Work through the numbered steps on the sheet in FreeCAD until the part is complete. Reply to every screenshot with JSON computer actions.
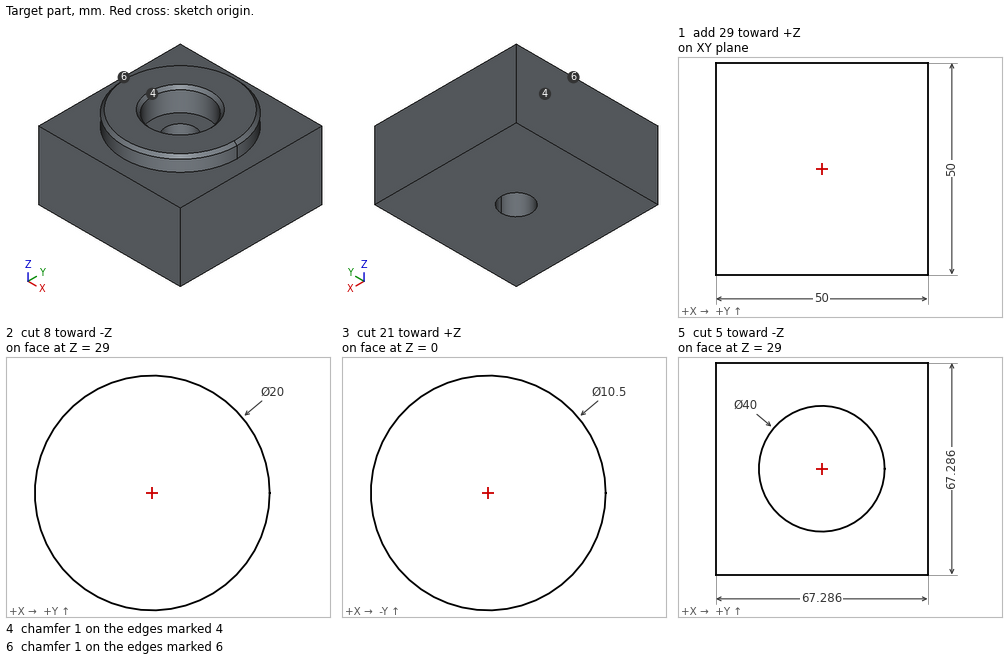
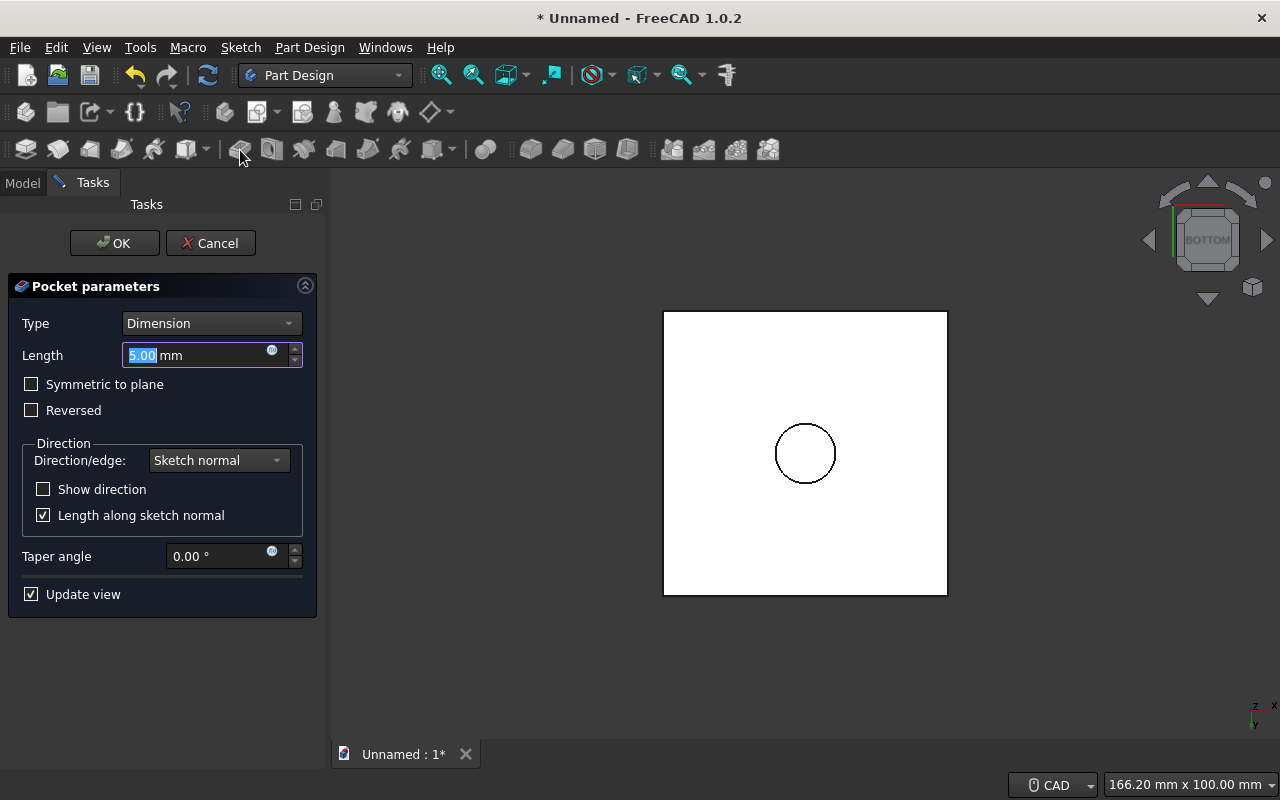
{"action": "type", "text": "21"}
{"action": "key", "text": "Tab"}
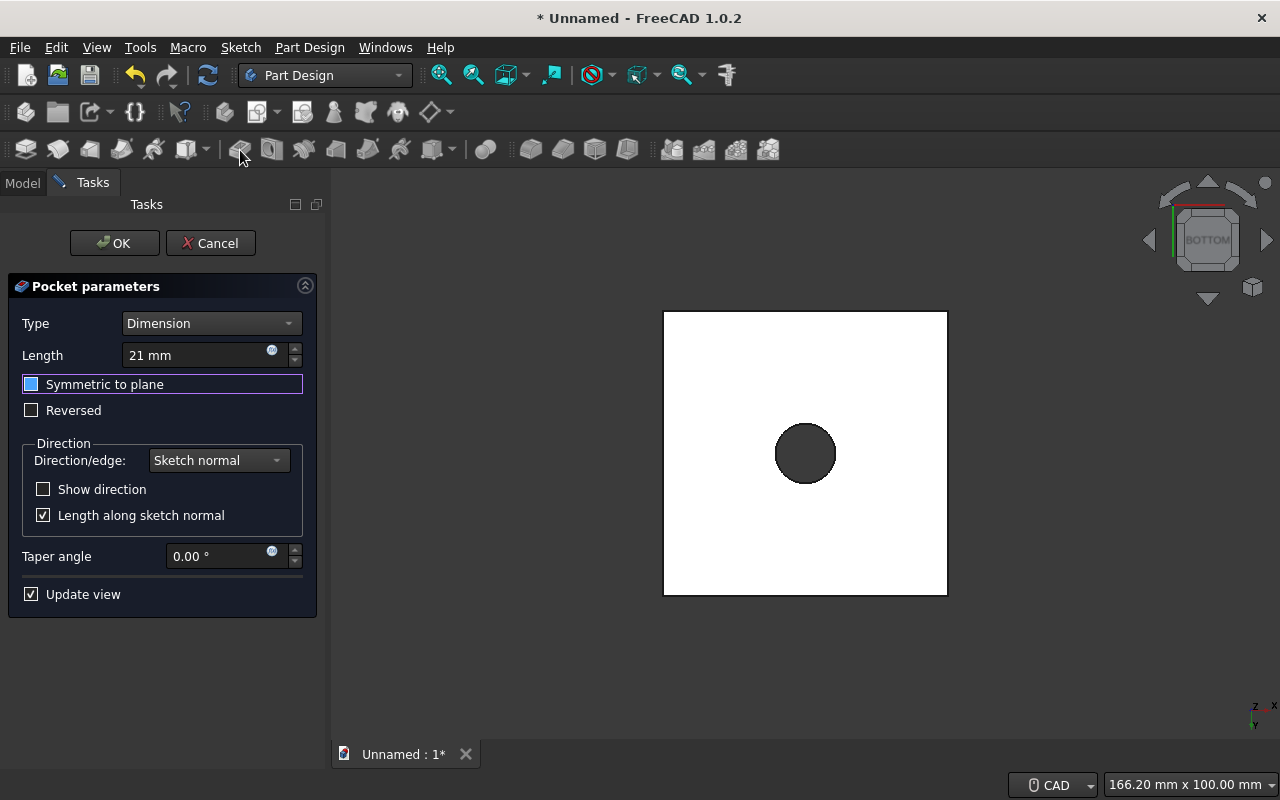
{"action": "left_click", "coordinate": [115, 243]}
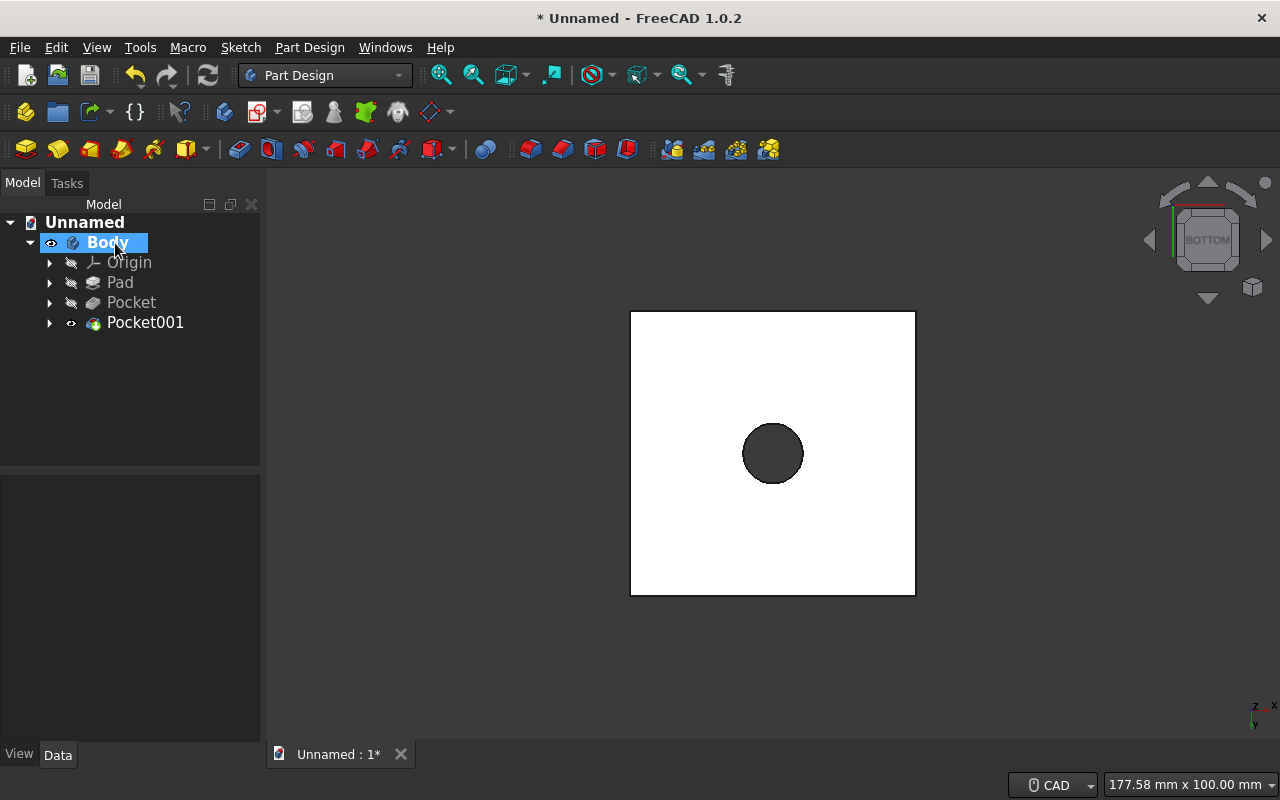
{"action": "key", "text": "0"}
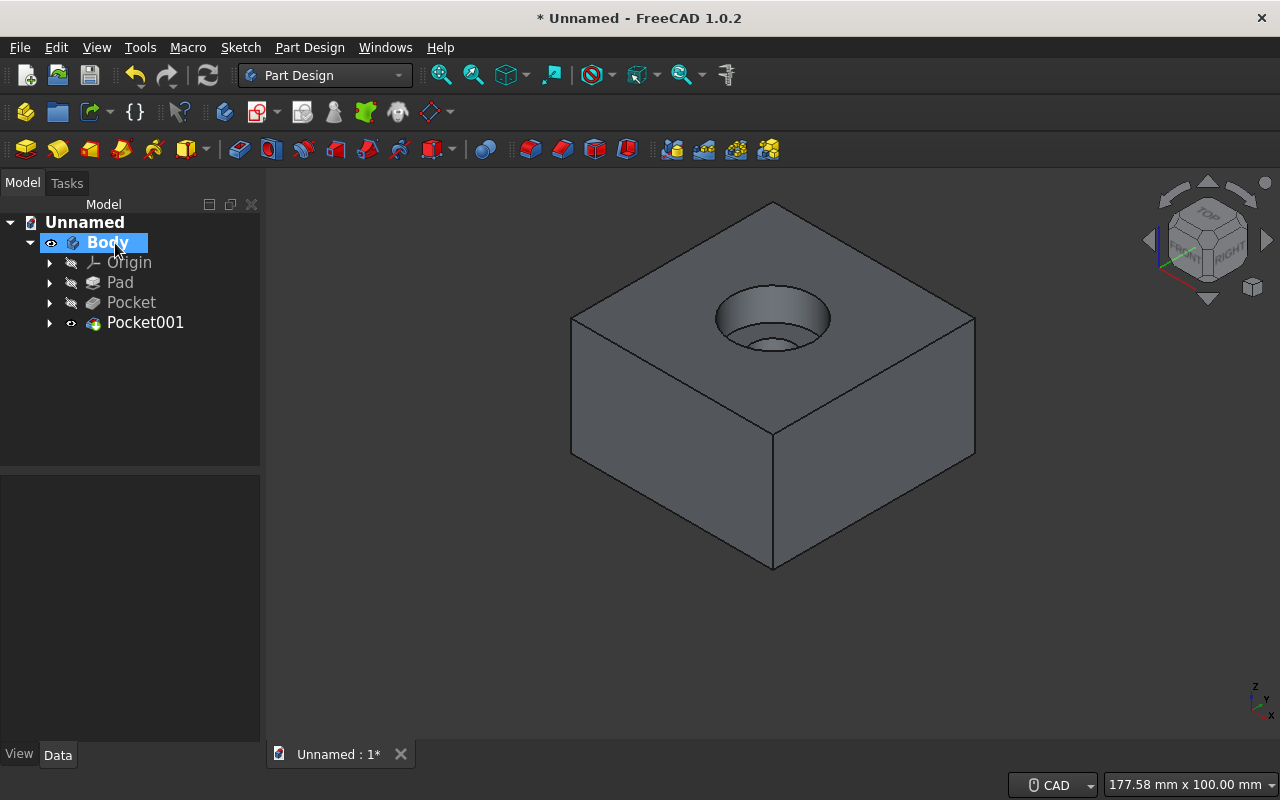
{"action": "left_click", "coordinate": [733, 294]}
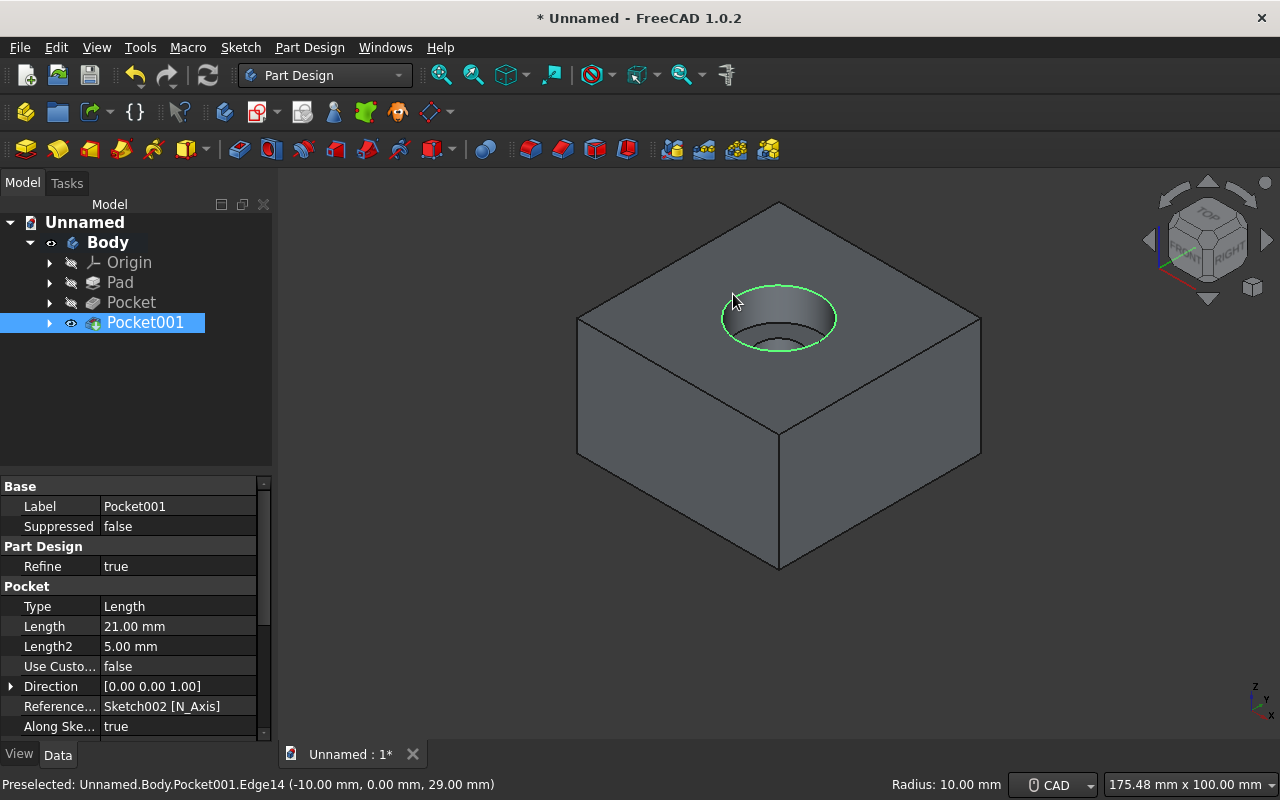
{"action": "left_click", "coordinate": [564, 150]}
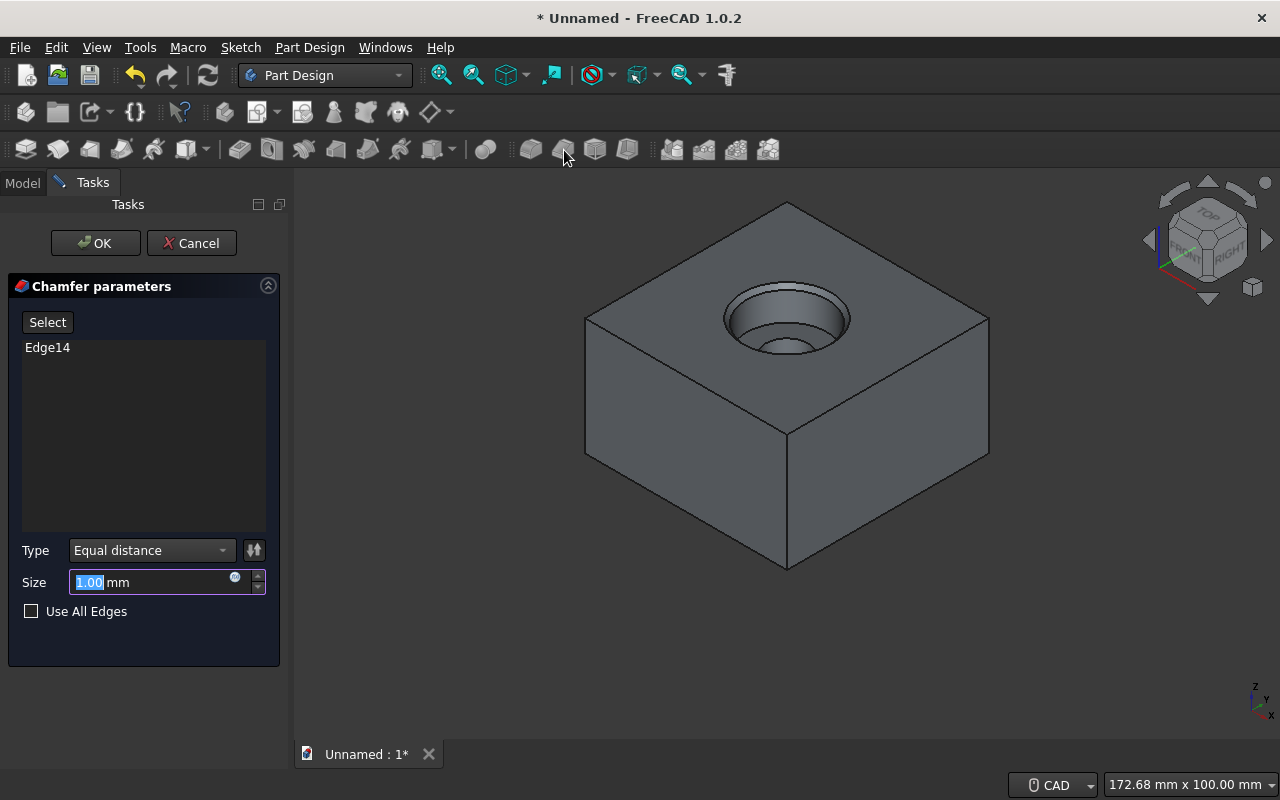
{"action": "type", "text": "1"}
{"action": "key", "text": "Tab"}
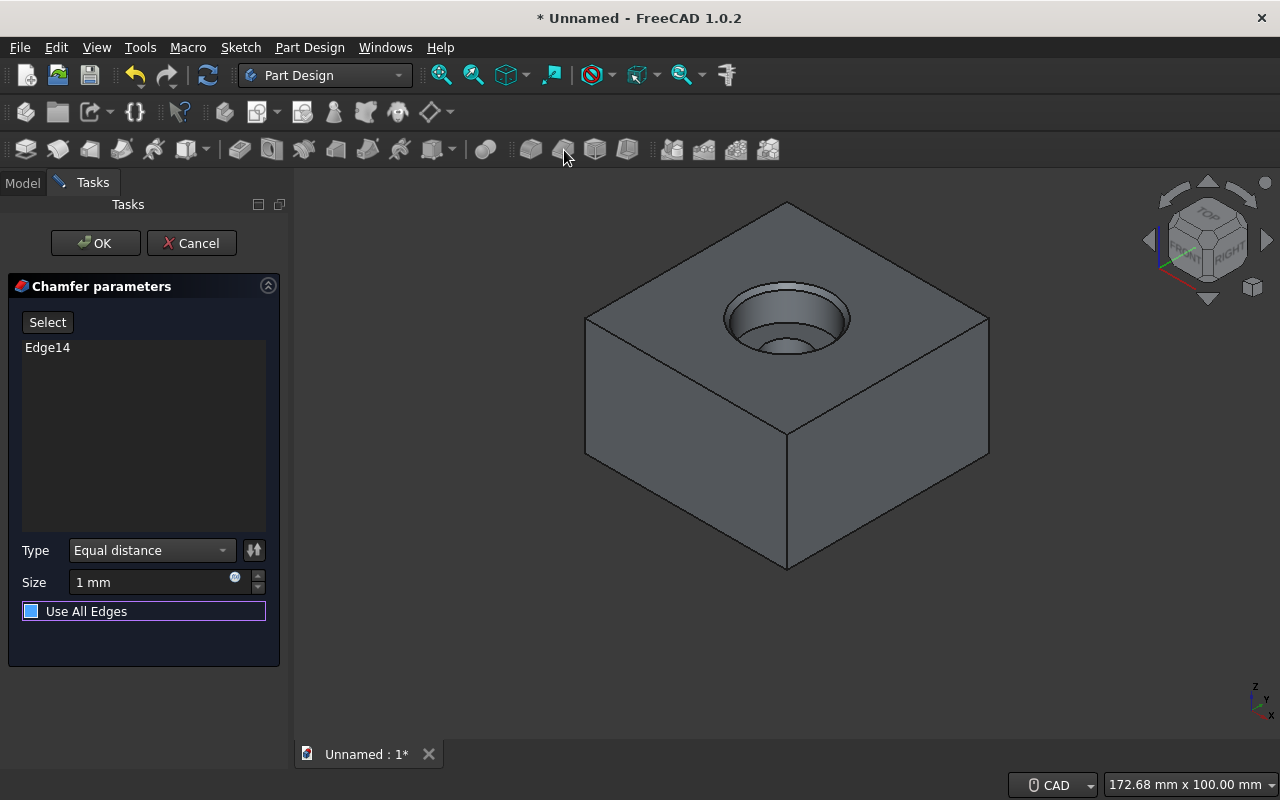
{"action": "left_click", "coordinate": [96, 243]}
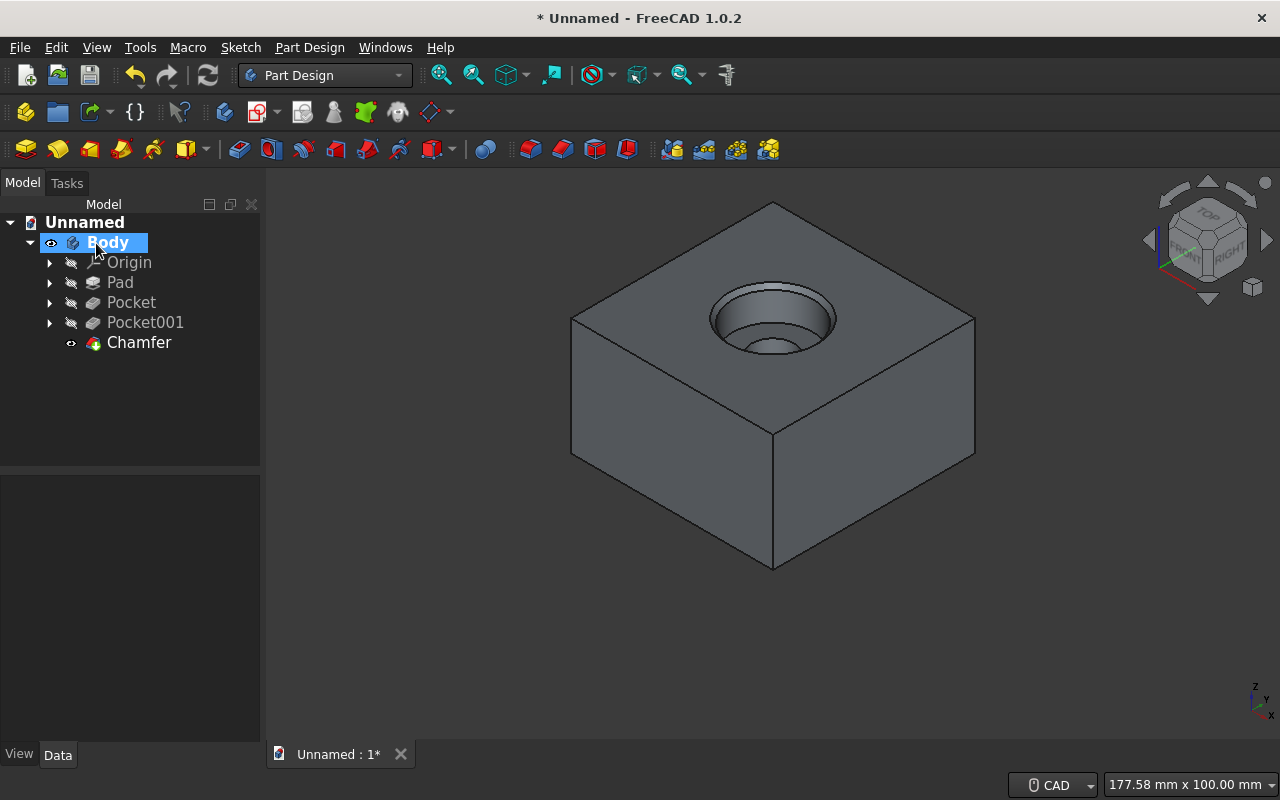
{"action": "left_click", "coordinate": [773, 251]}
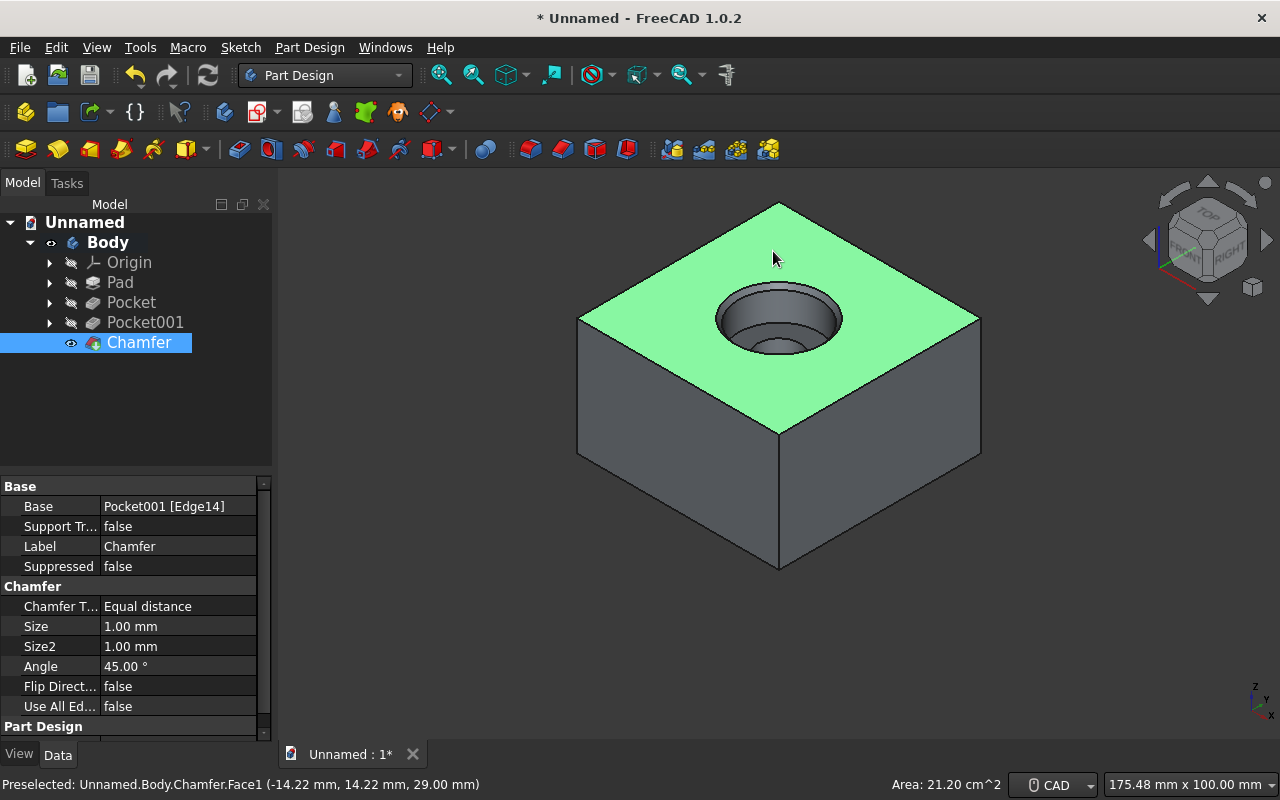
{"action": "left_click", "coordinate": [258, 112]}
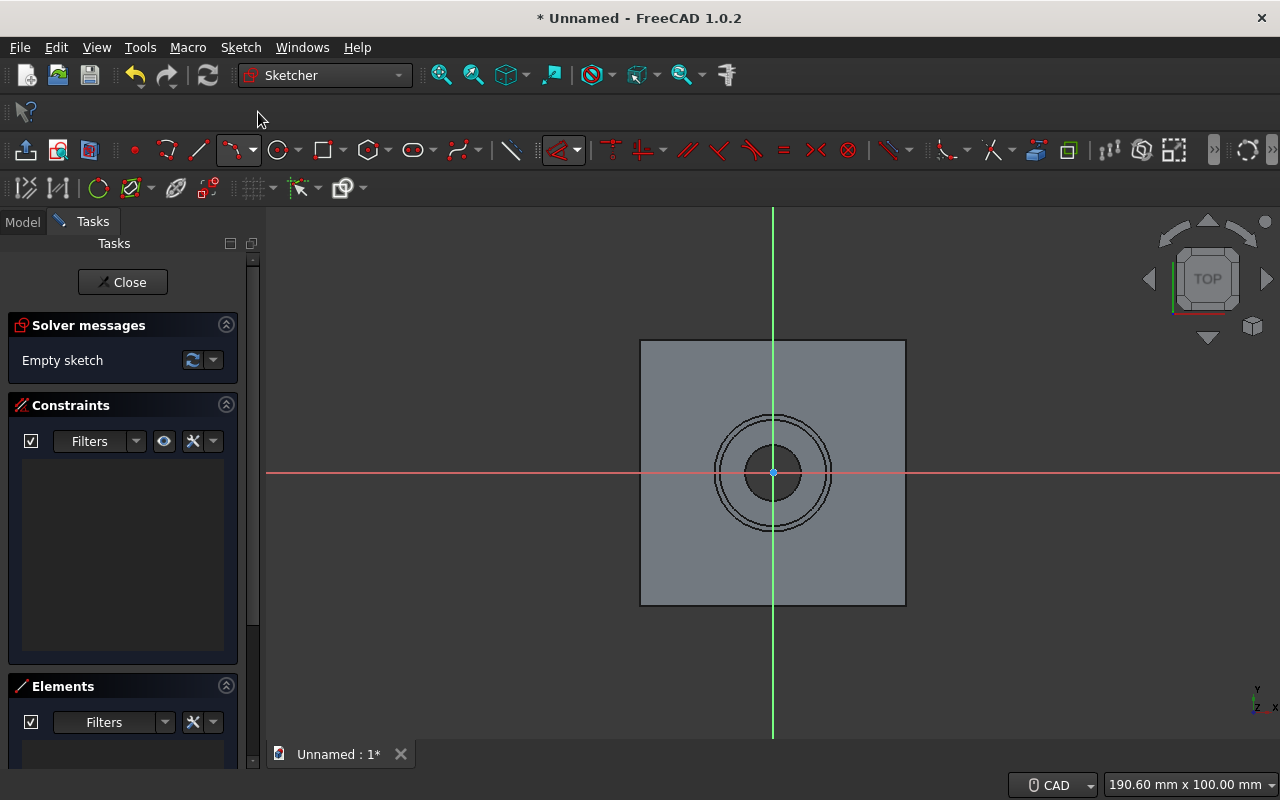
{"action": "key", "text": "g v"}